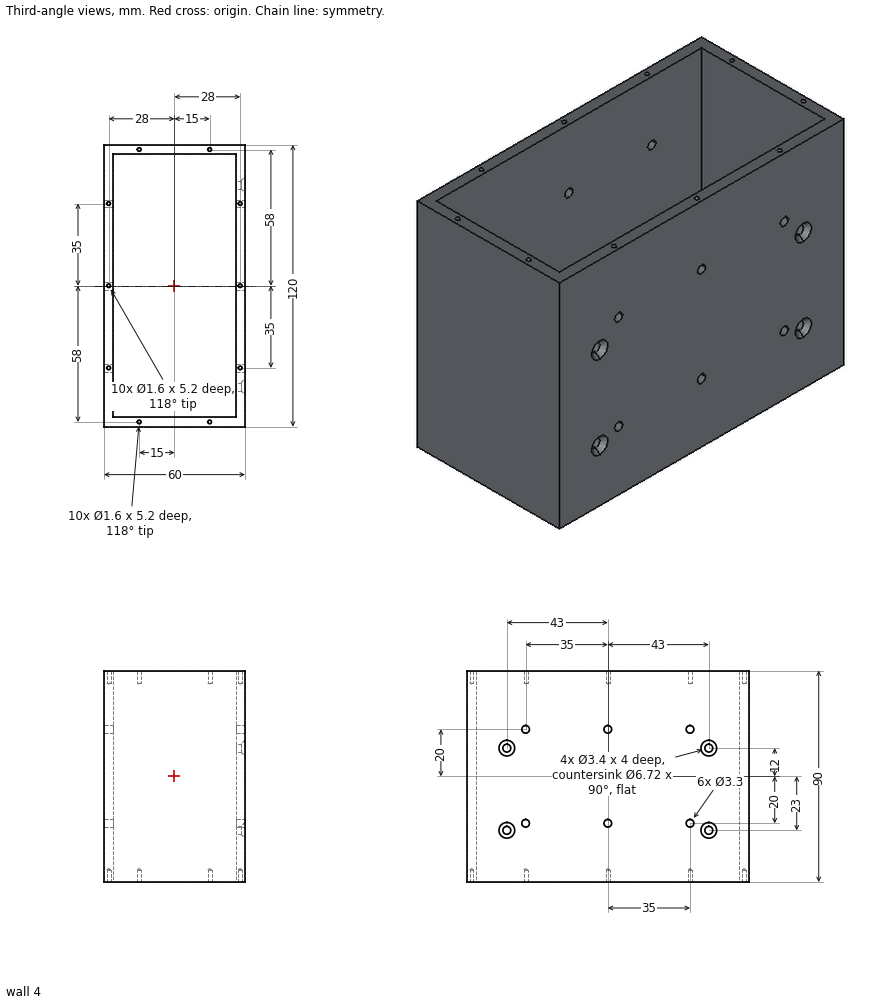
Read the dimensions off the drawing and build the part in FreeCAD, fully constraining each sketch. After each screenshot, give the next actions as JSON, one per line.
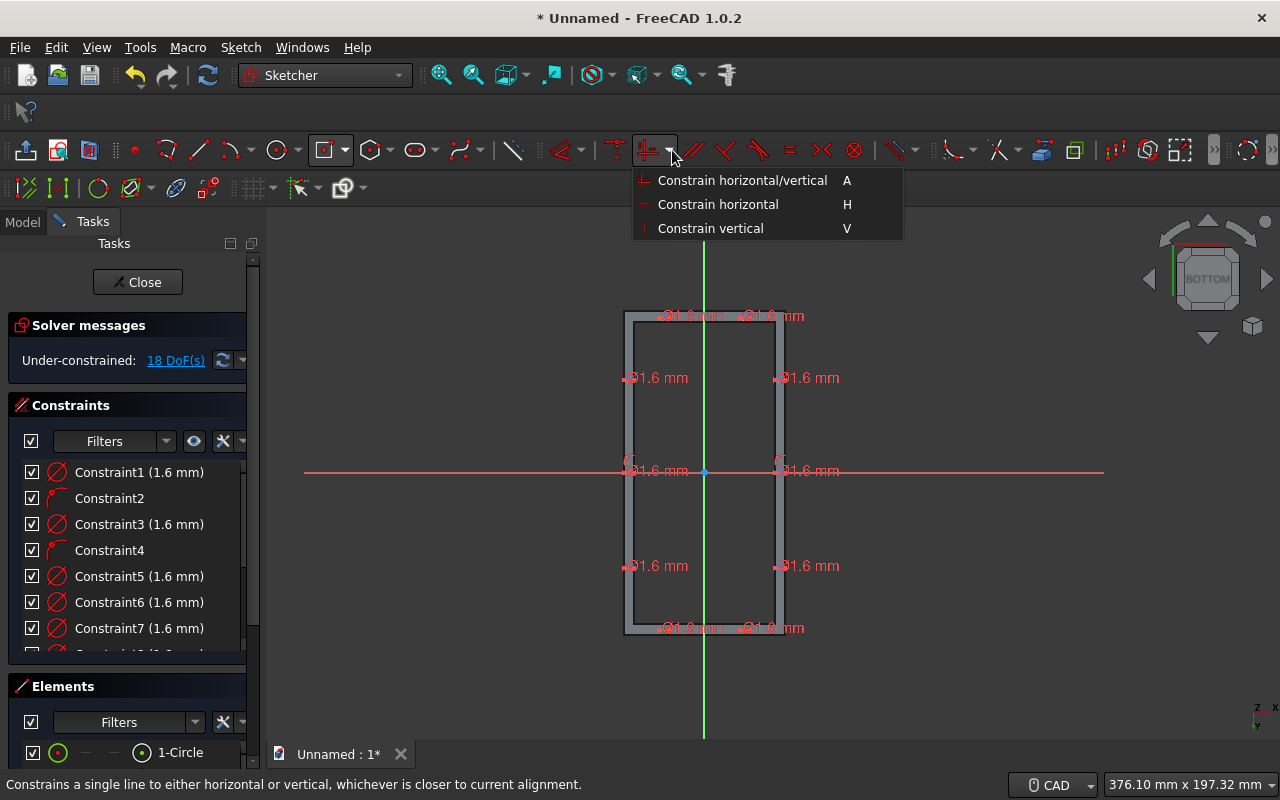
{"action": "left_click", "coordinate": [768, 204]}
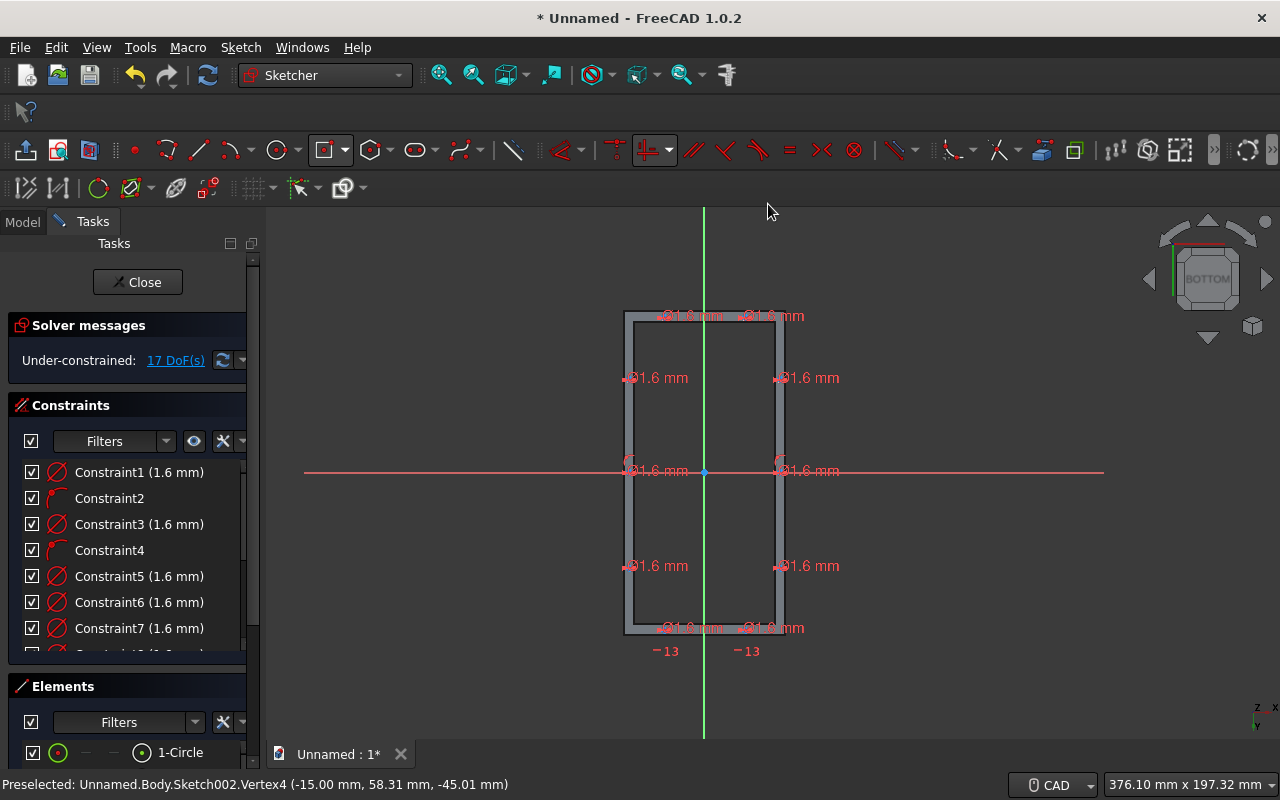
{"action": "left_click", "coordinate": [629, 473]}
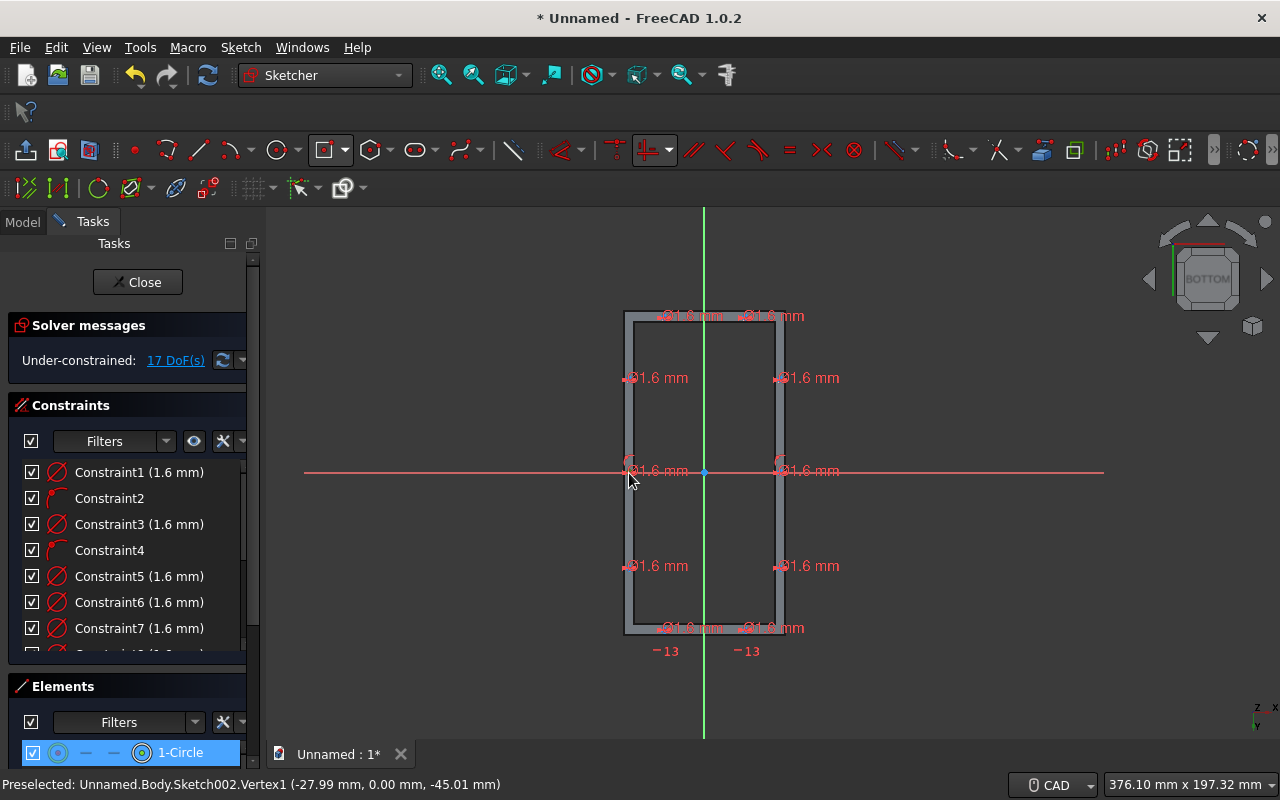
{"action": "left_click", "coordinate": [629, 568]}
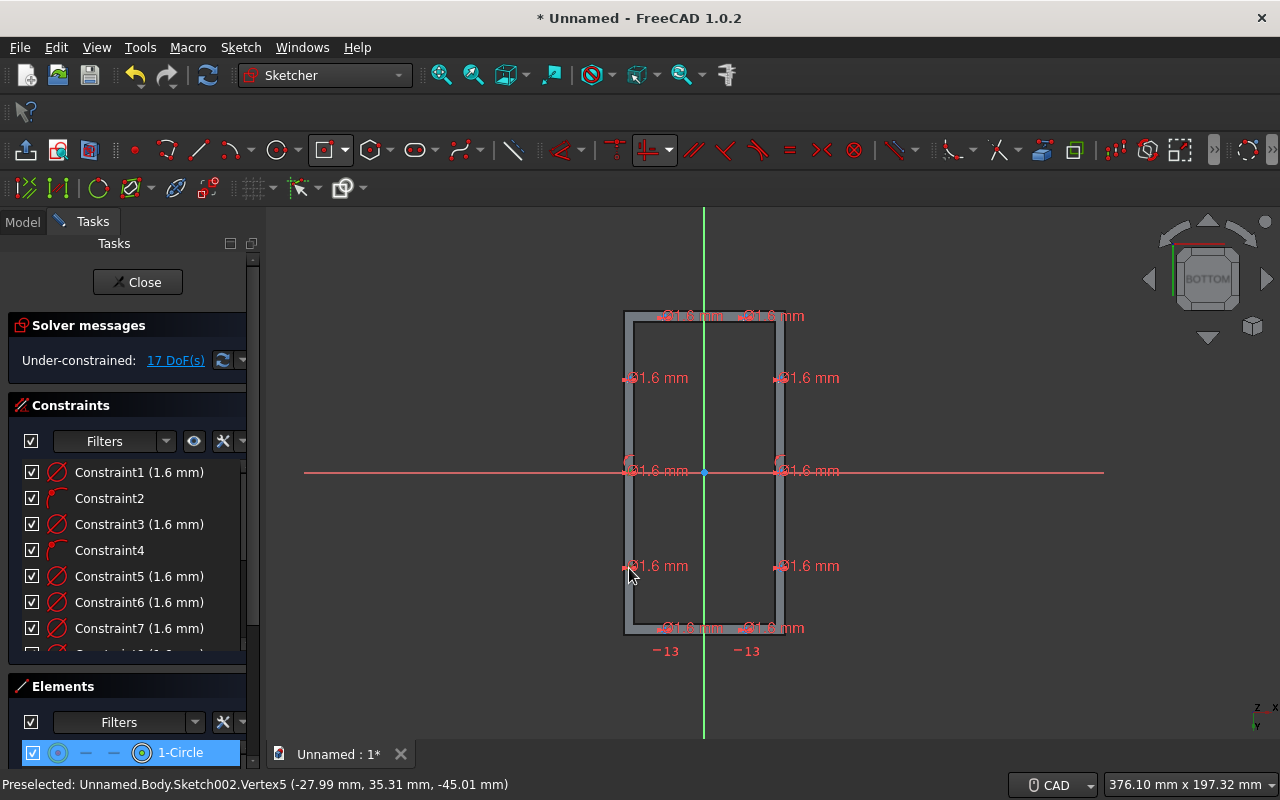
{"action": "left_click", "coordinate": [672, 150]}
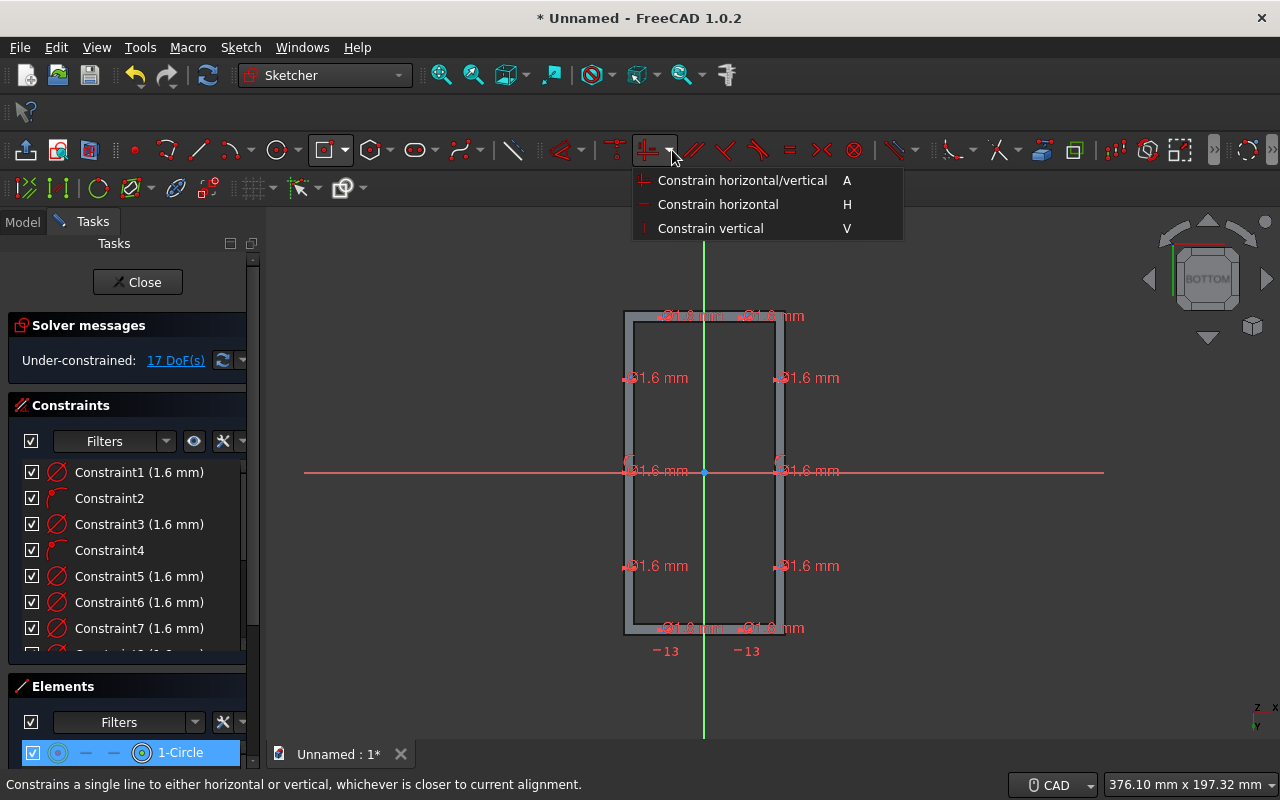
{"action": "left_click", "coordinate": [768, 228]}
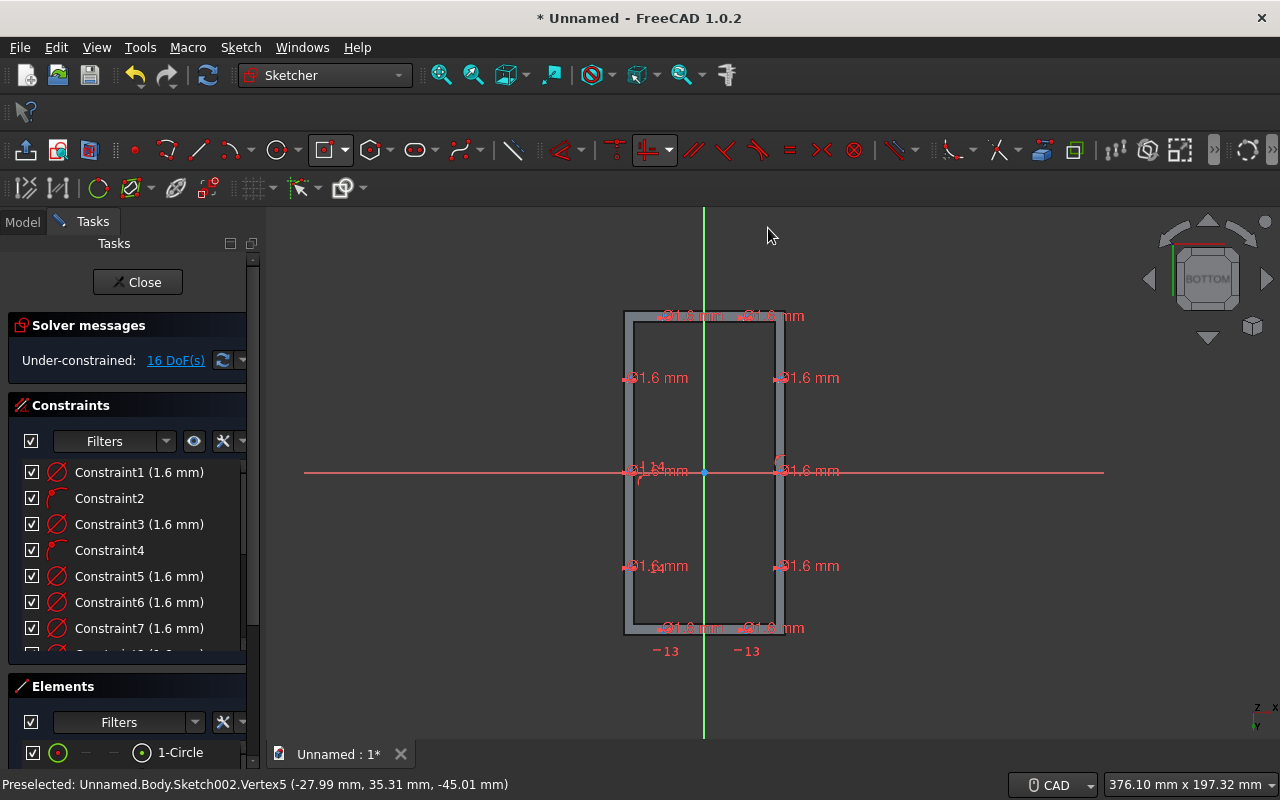
{"action": "left_click", "coordinate": [780, 473]}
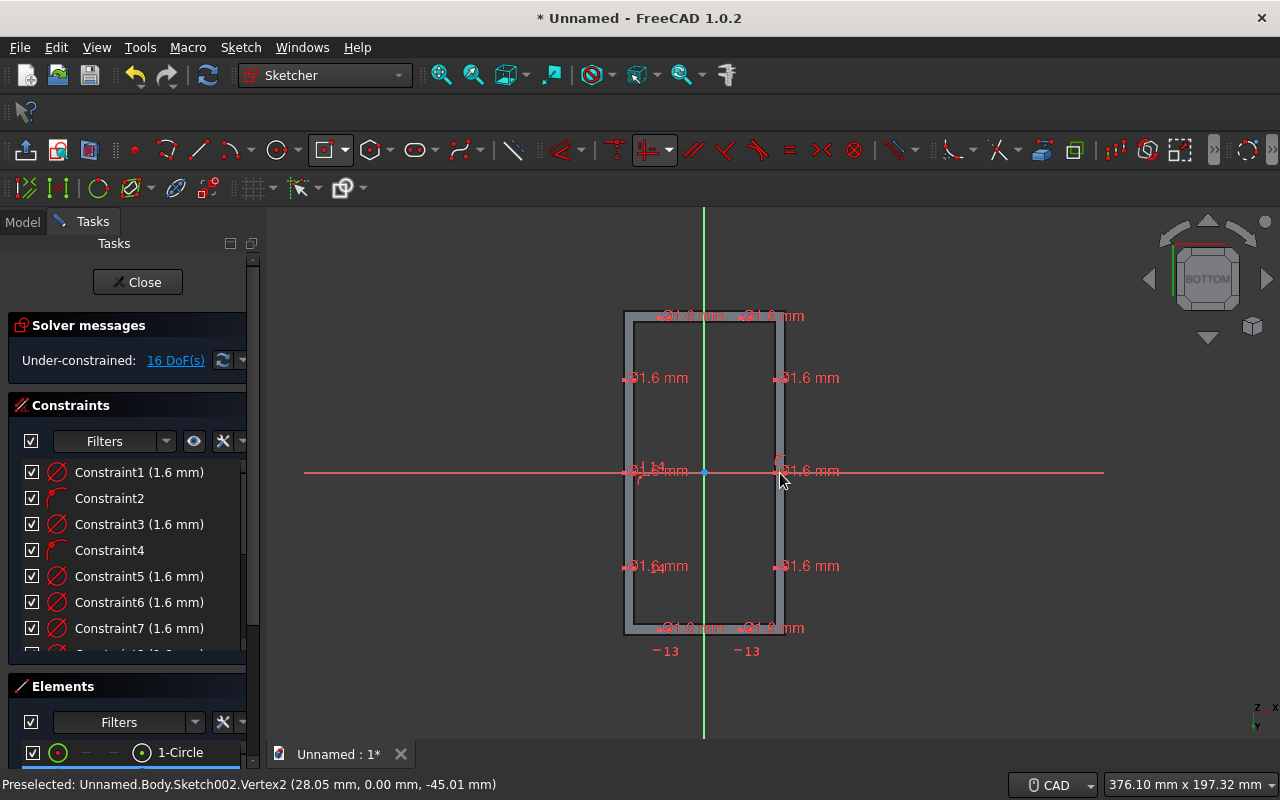
{"action": "left_click", "coordinate": [780, 568]}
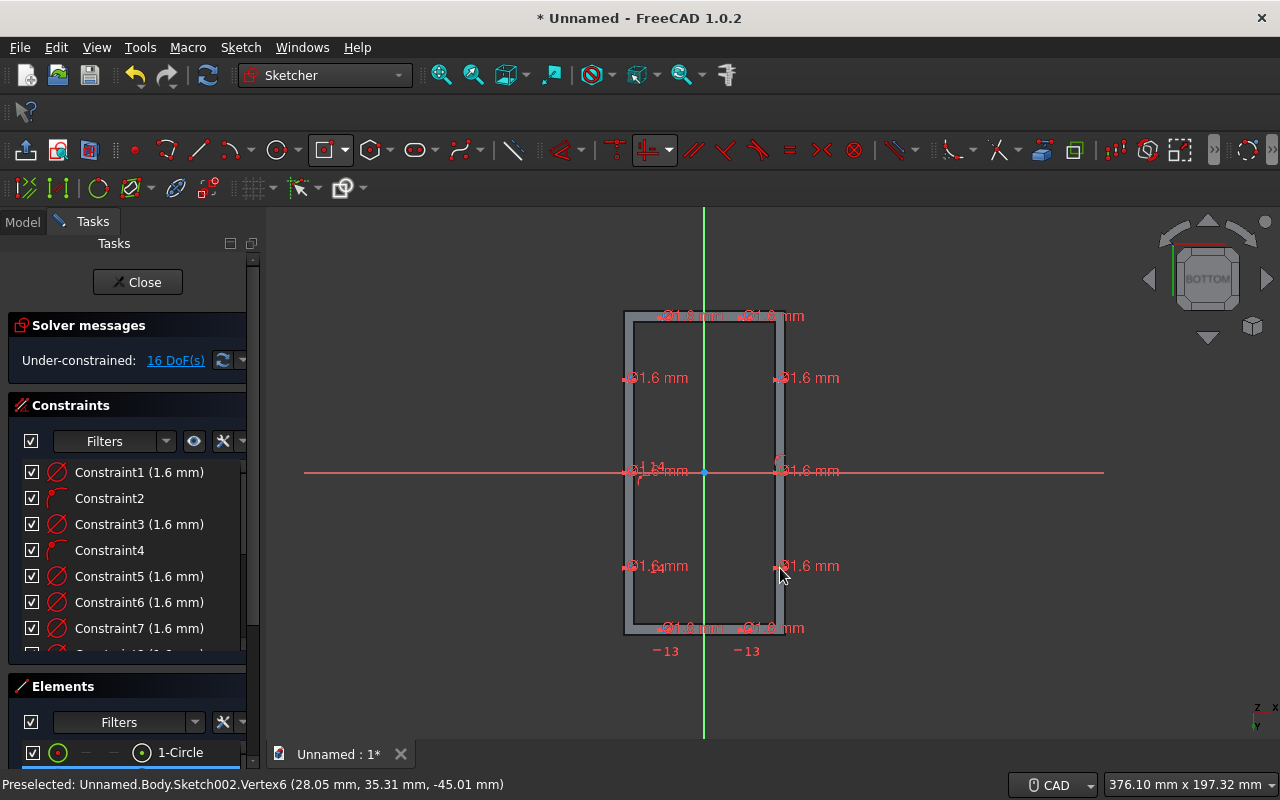
{"action": "key", "text": "v"}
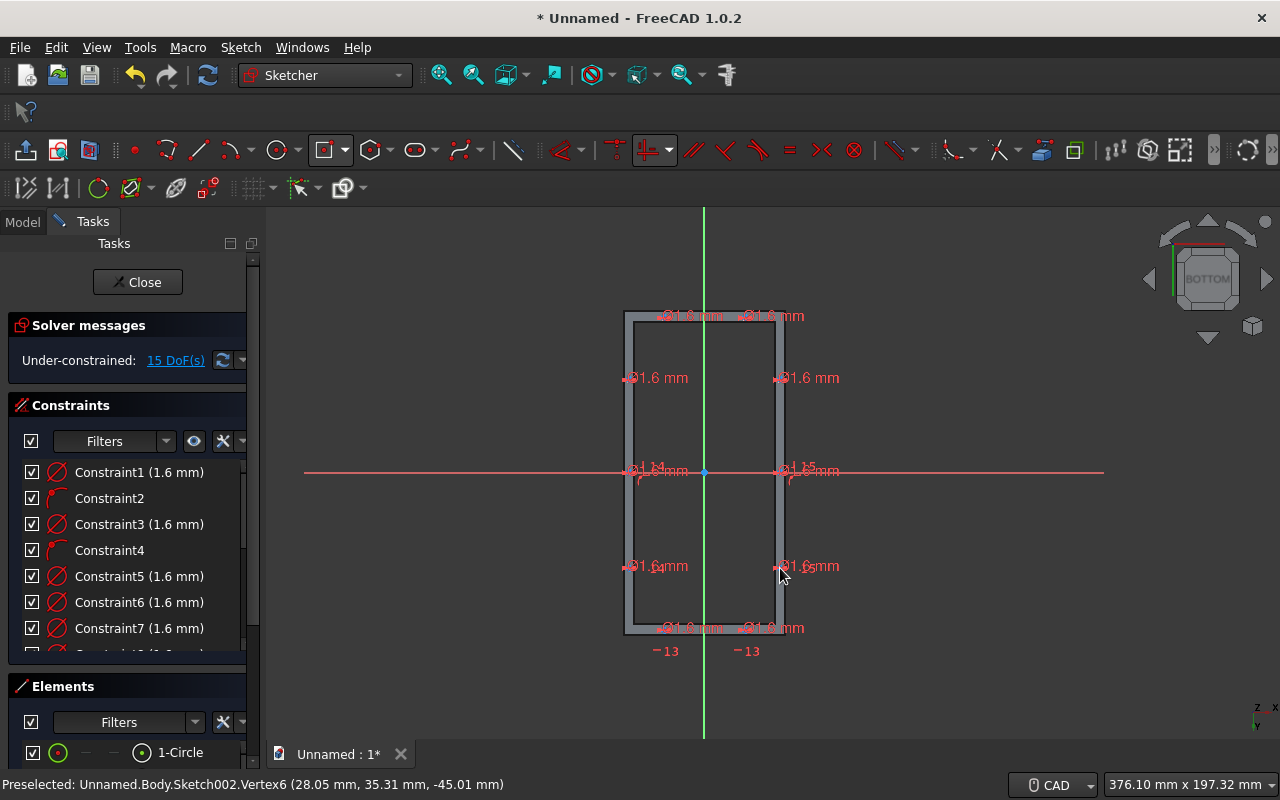
{"action": "left_click", "coordinate": [629, 568]}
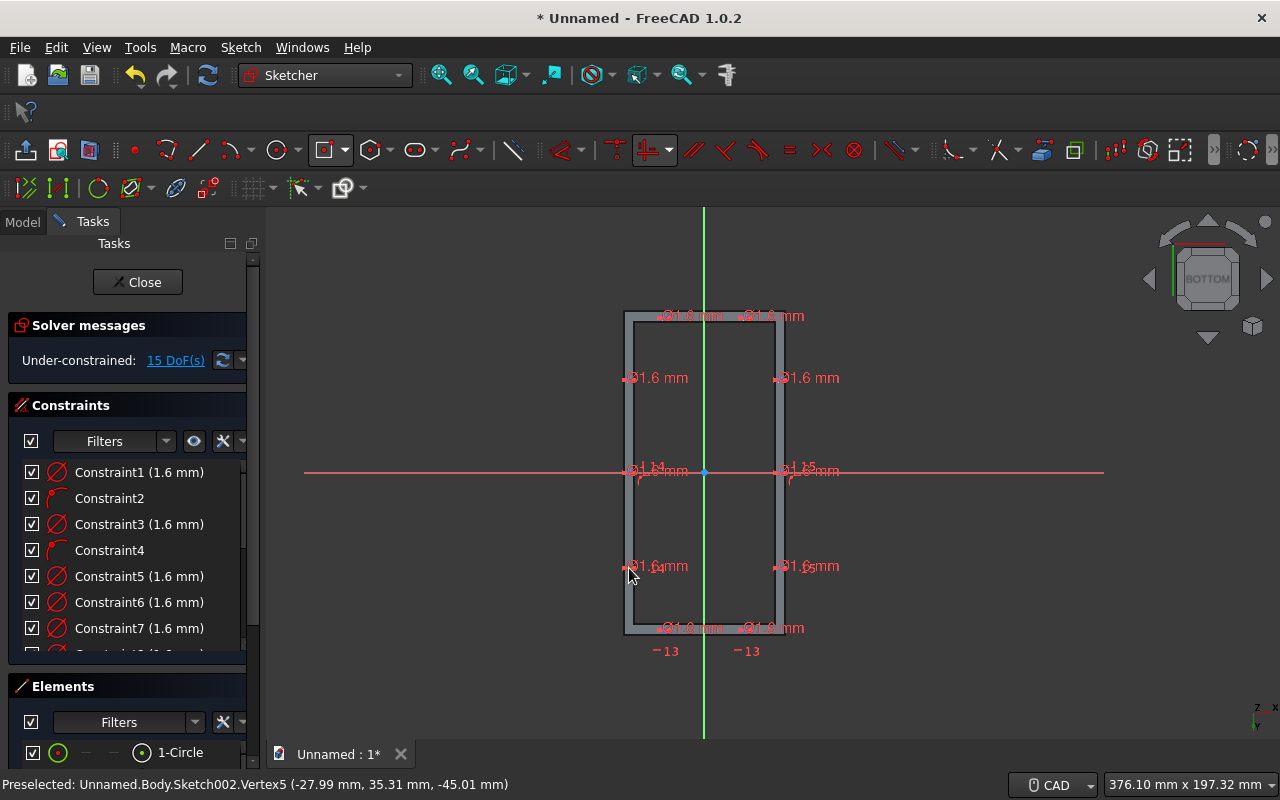
{"action": "left_click", "coordinate": [780, 568]}